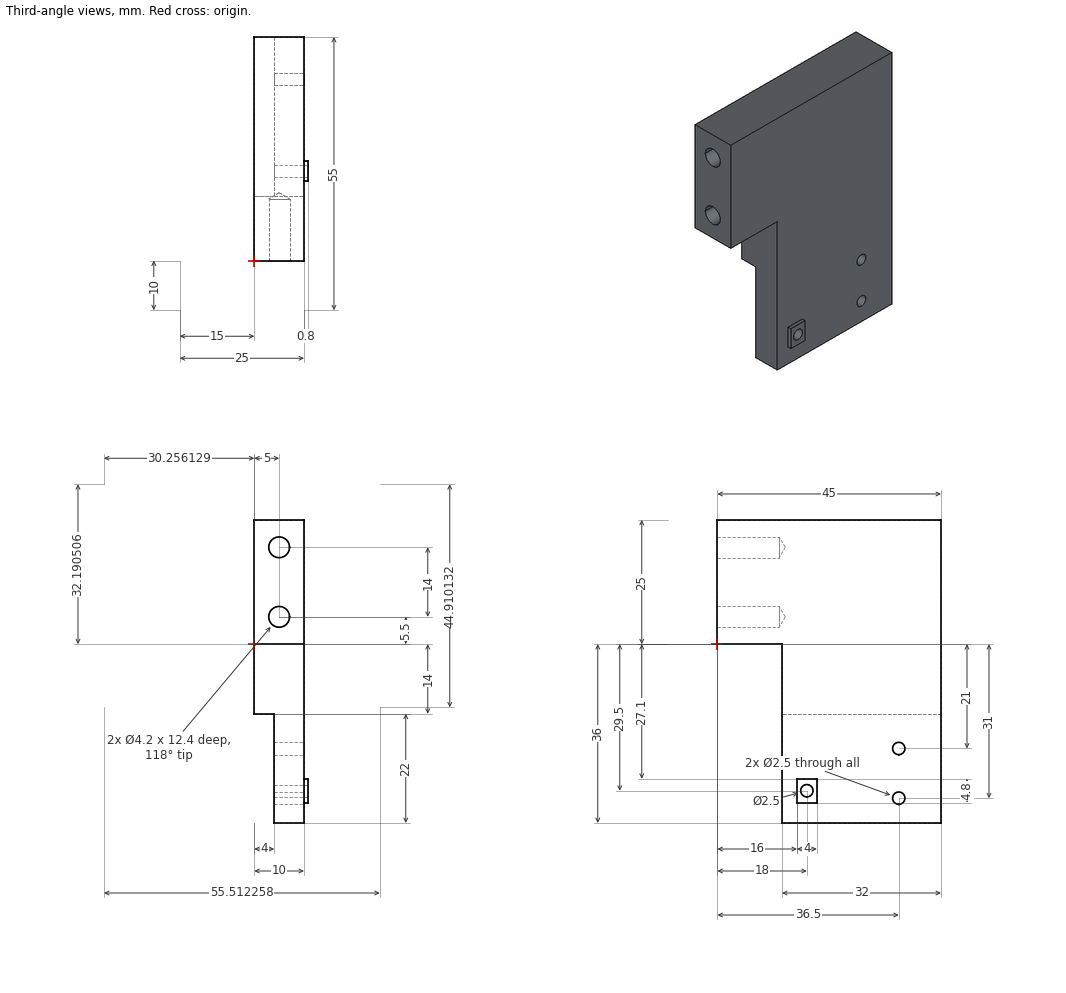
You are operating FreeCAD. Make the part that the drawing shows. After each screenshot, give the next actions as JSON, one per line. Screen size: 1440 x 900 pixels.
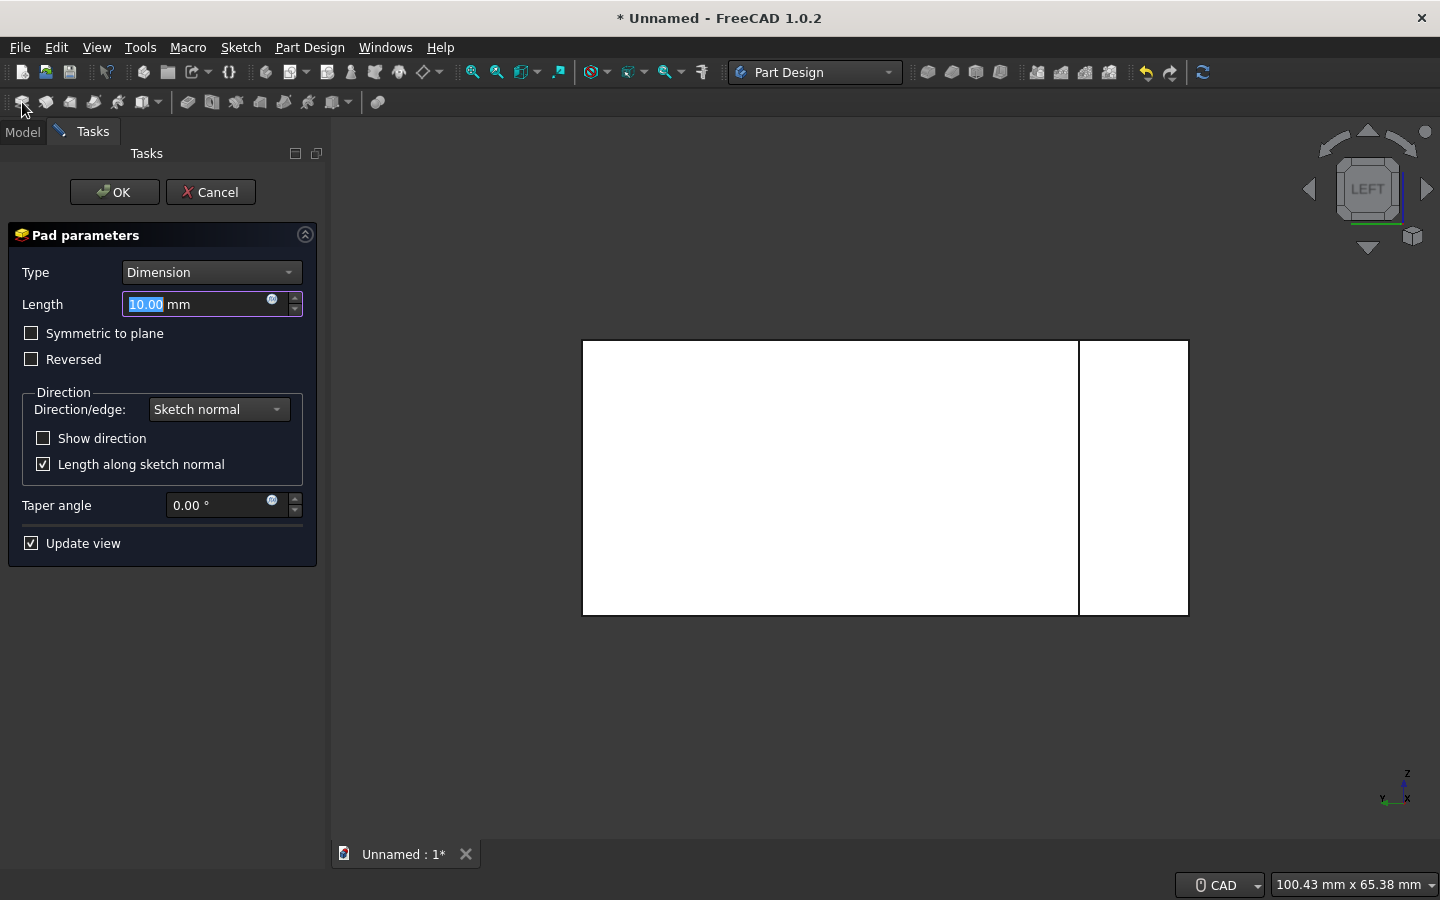
{"action": "type", "text": "10"}
{"action": "key", "text": "Tab"}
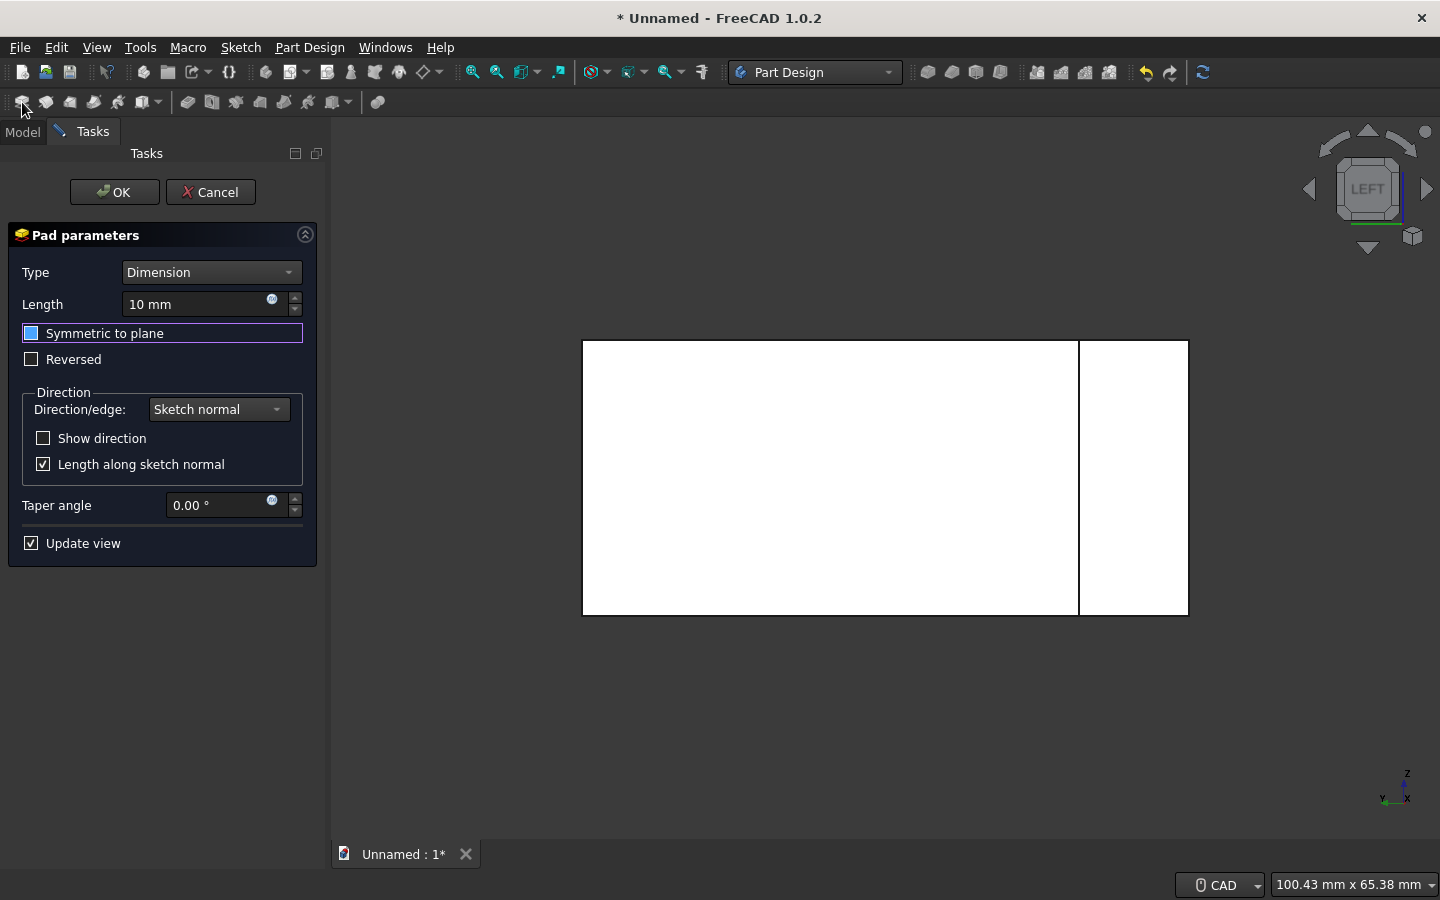
{"action": "left_click", "coordinate": [30, 359]}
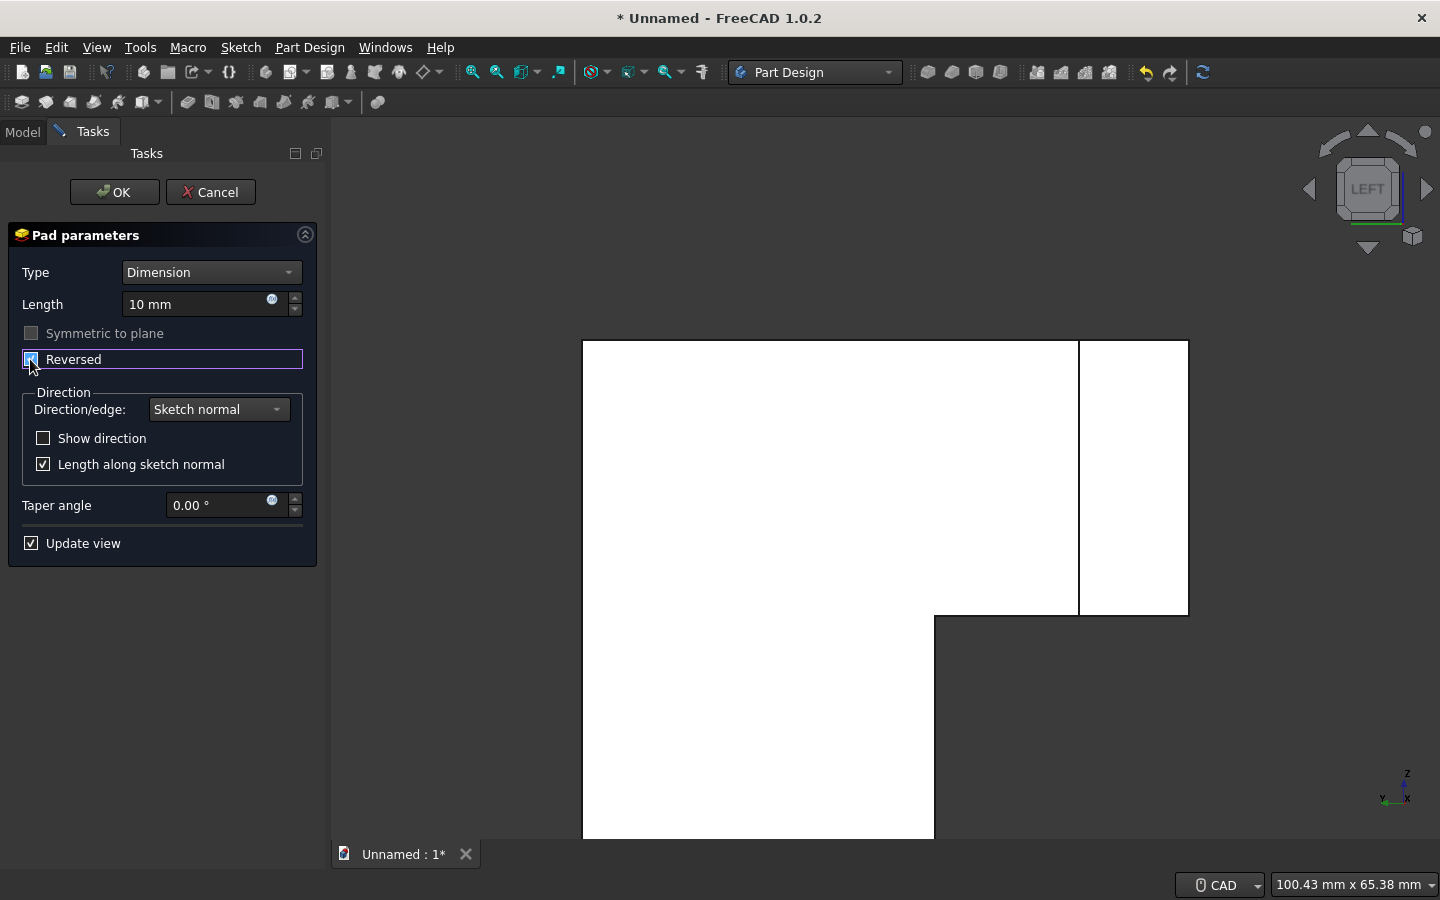
{"action": "left_click", "coordinate": [115, 192]}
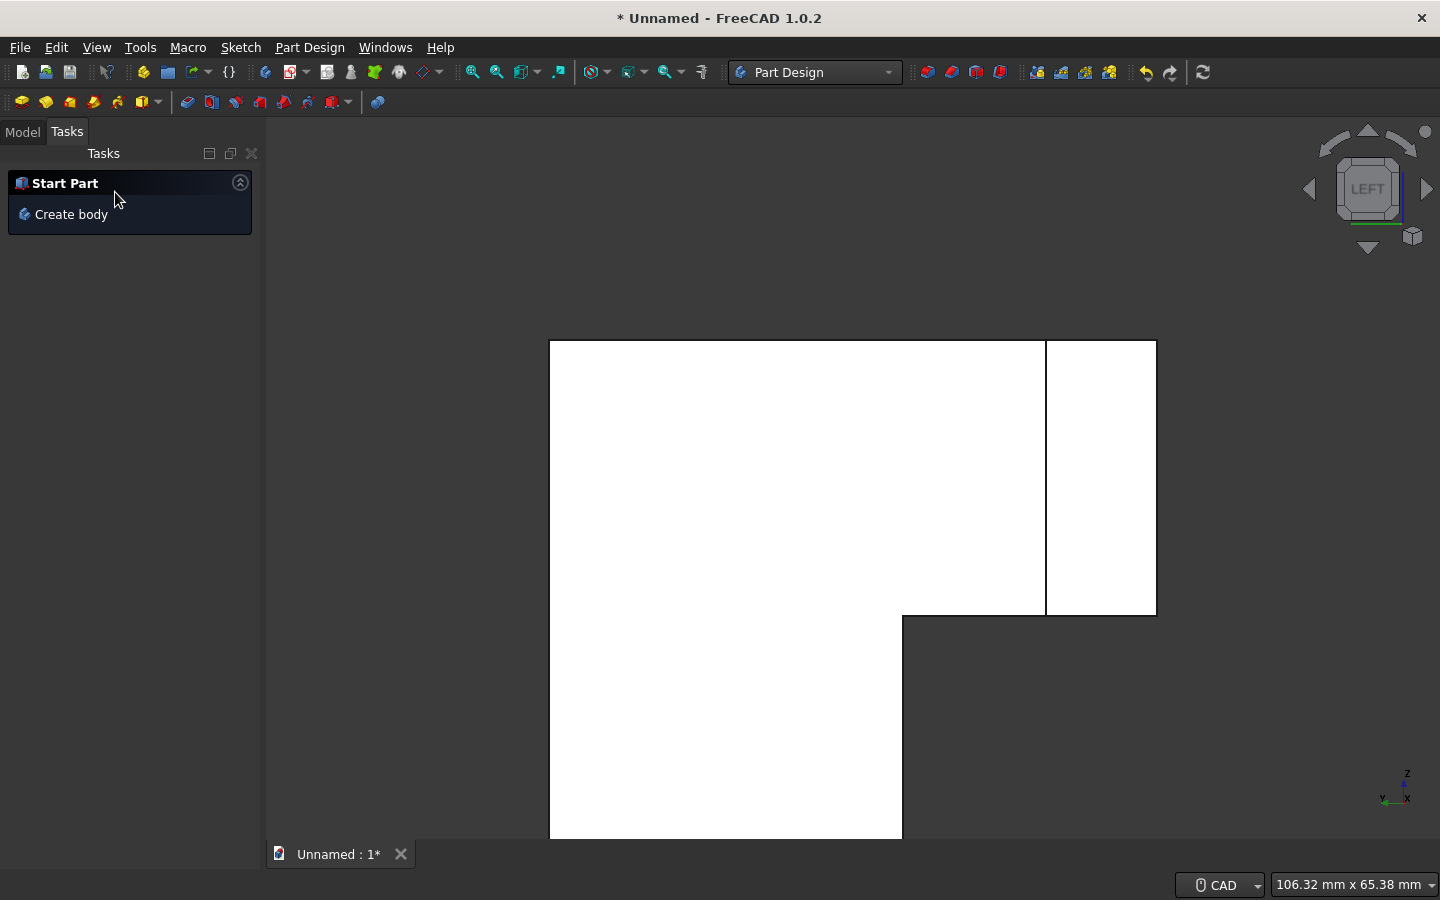
{"action": "key", "text": "v f"}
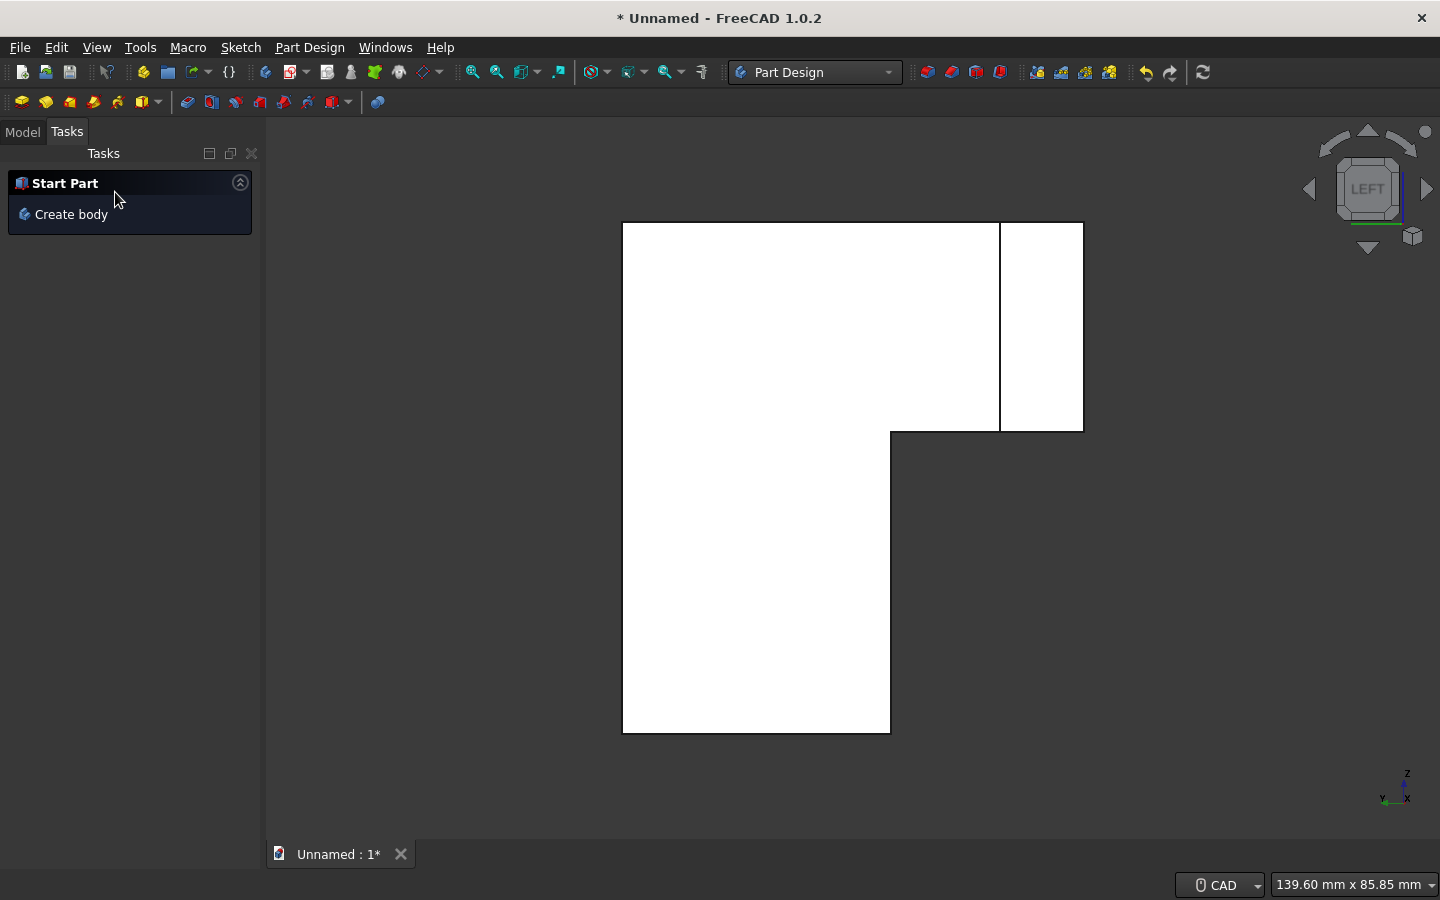
{"action": "key", "text": "4"}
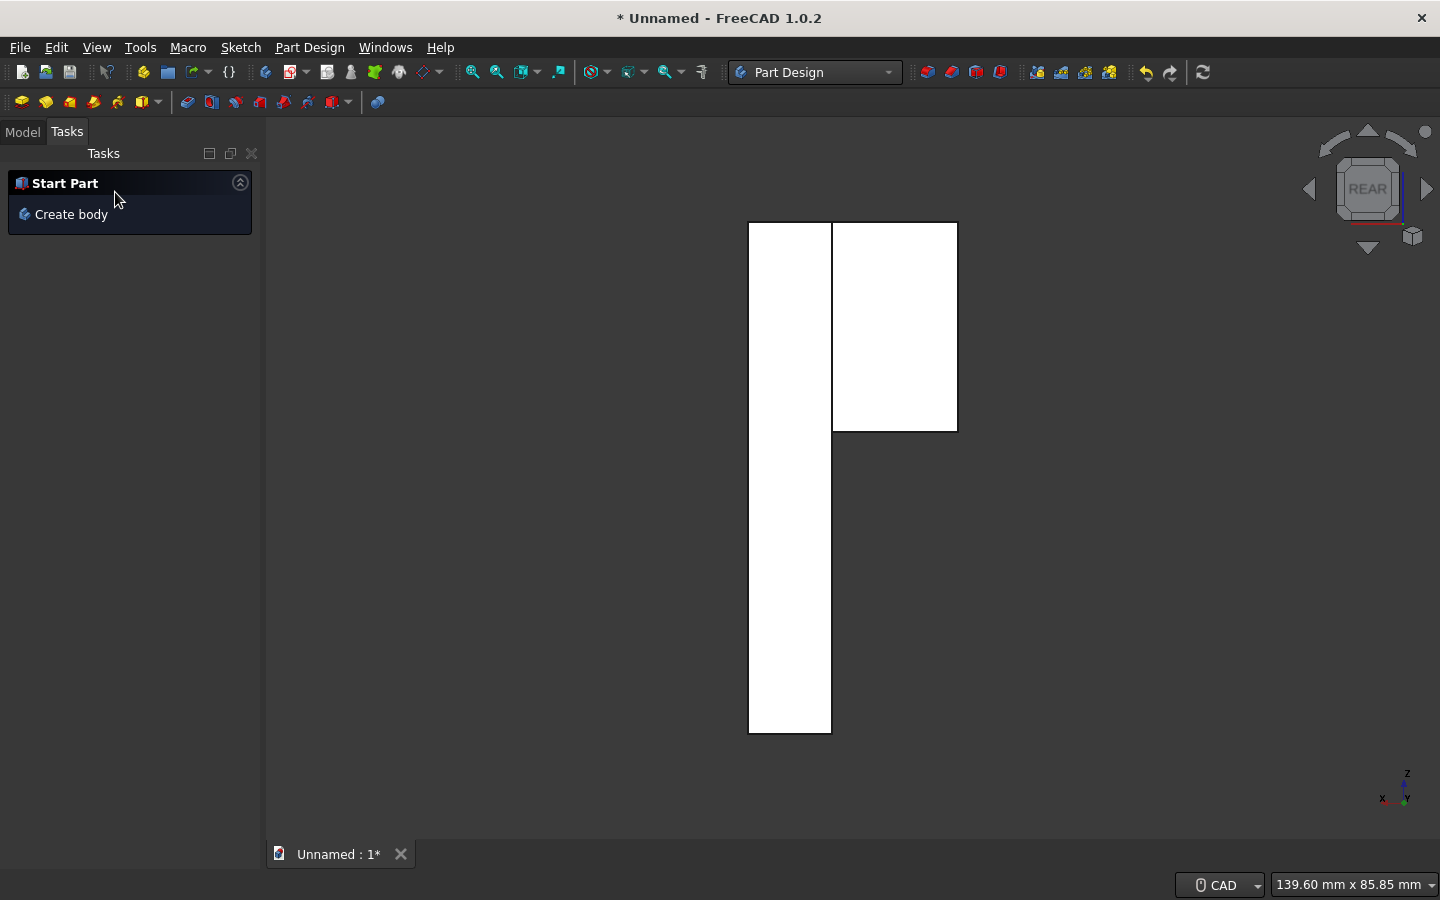
{"action": "left_click", "coordinate": [790, 330]}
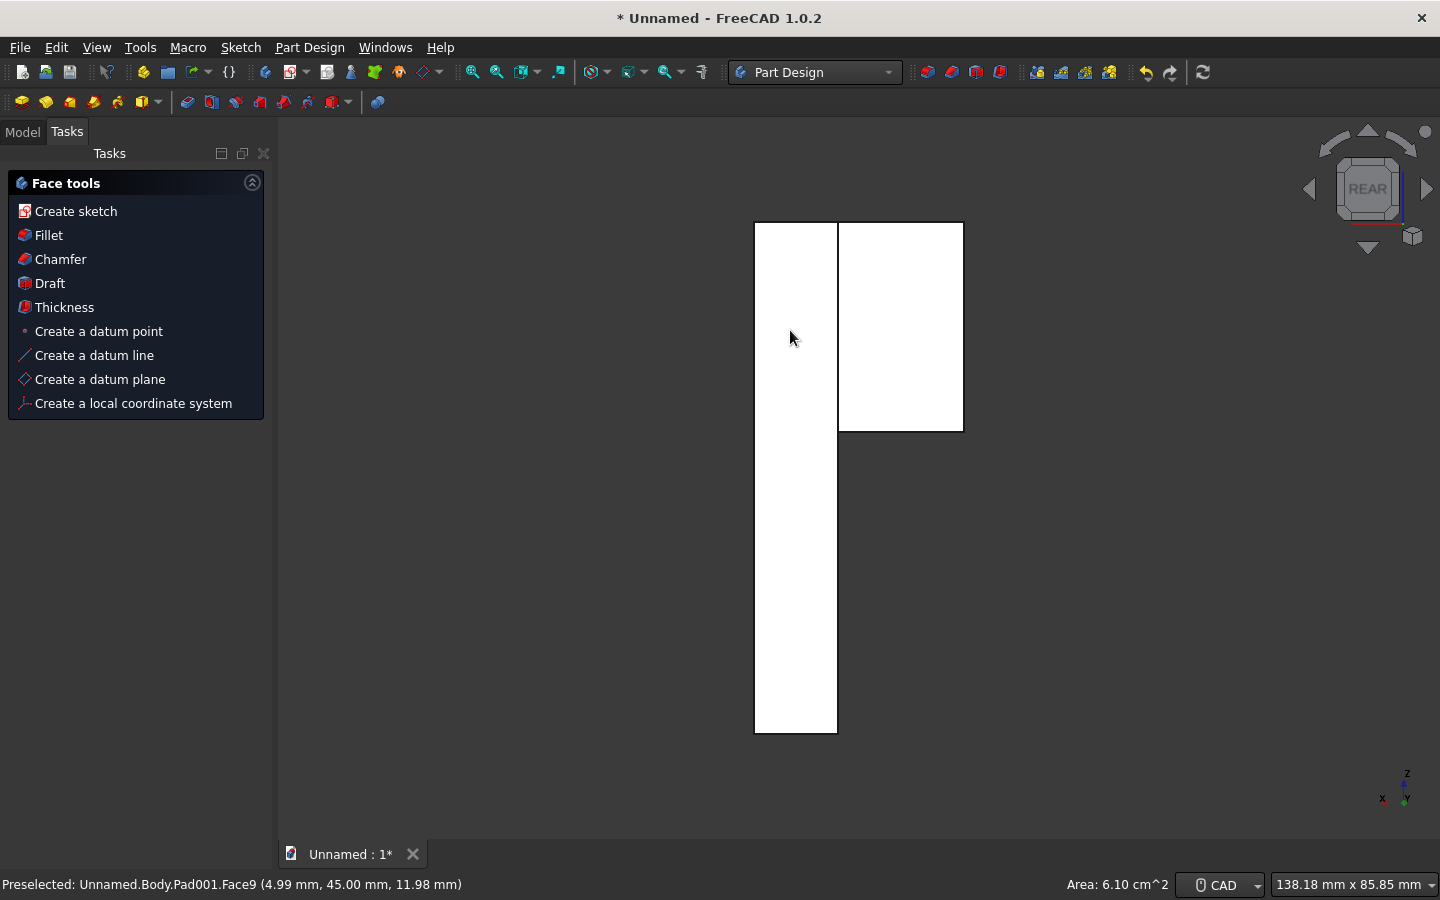
{"action": "left_click", "coordinate": [290, 72]}